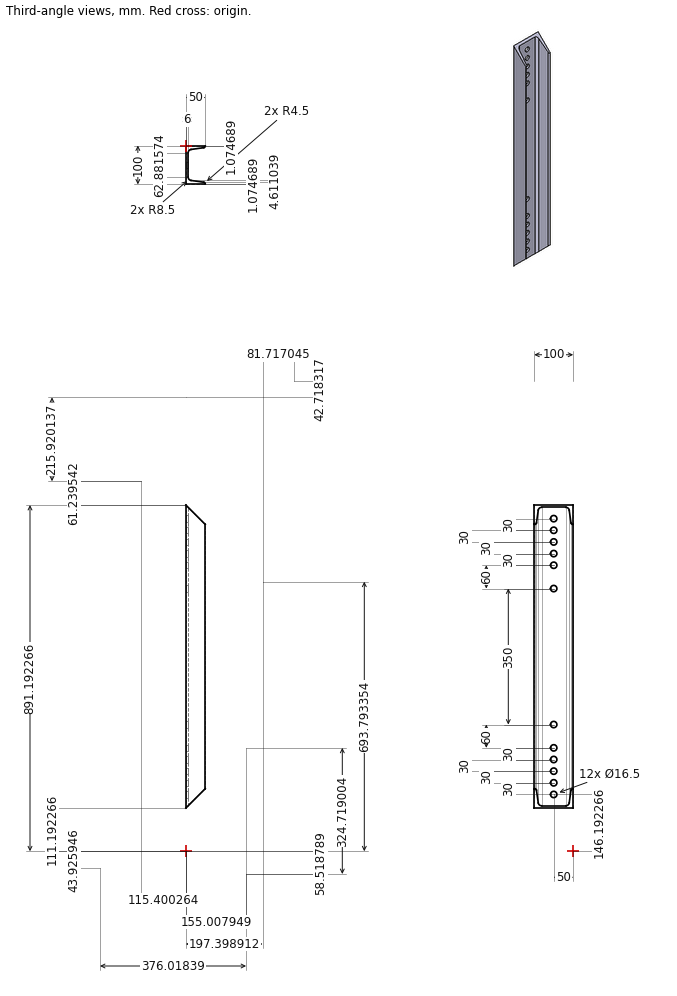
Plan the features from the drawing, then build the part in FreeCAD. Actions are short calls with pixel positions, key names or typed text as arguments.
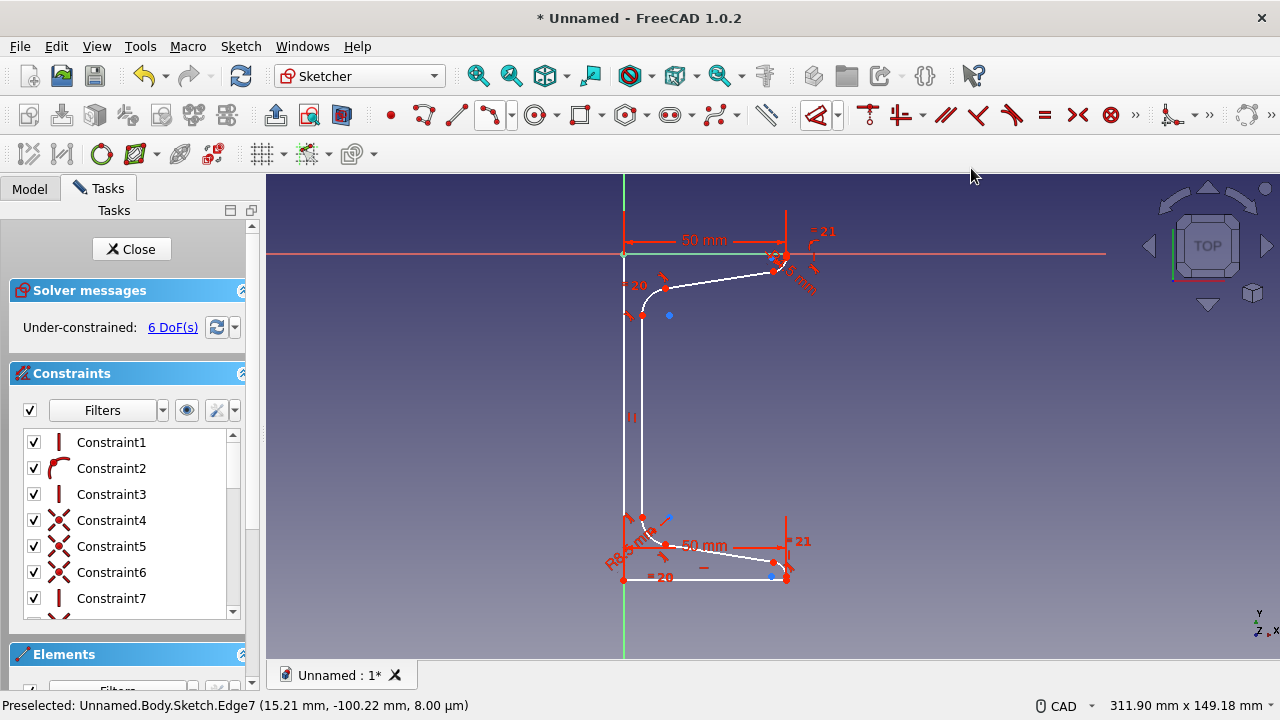
scroll(642, 518, up, 4)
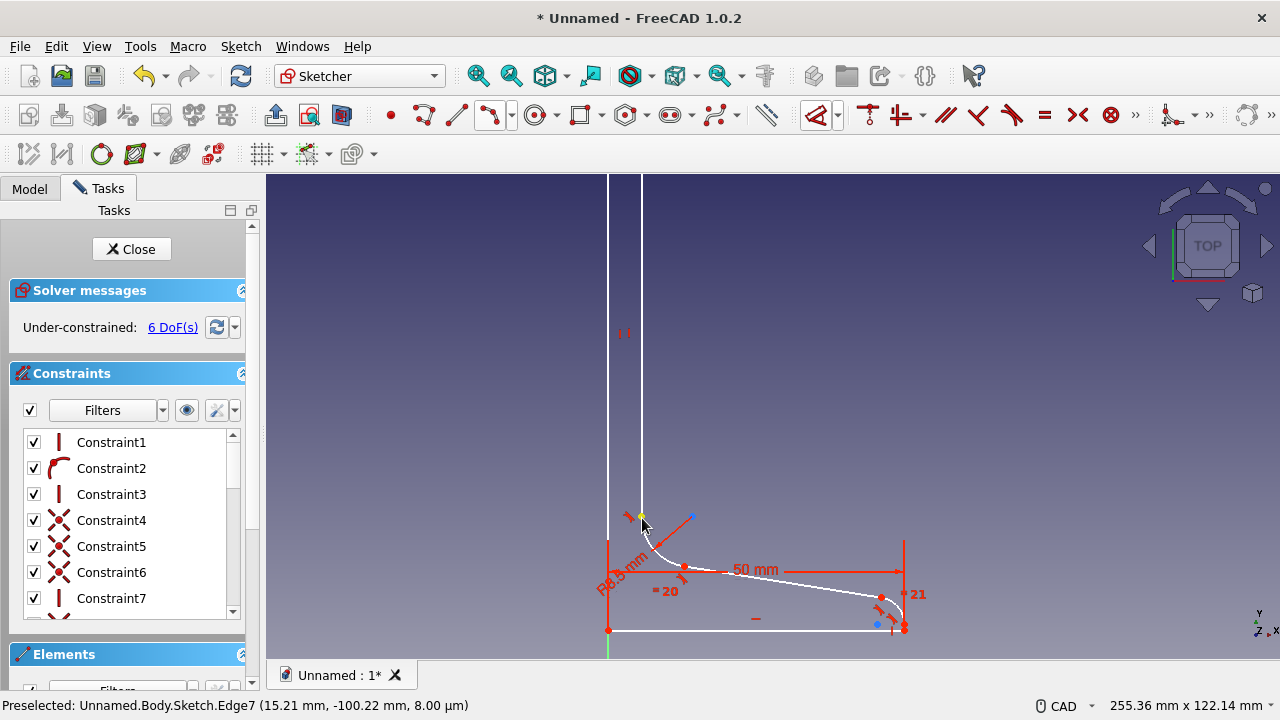
click(642, 516)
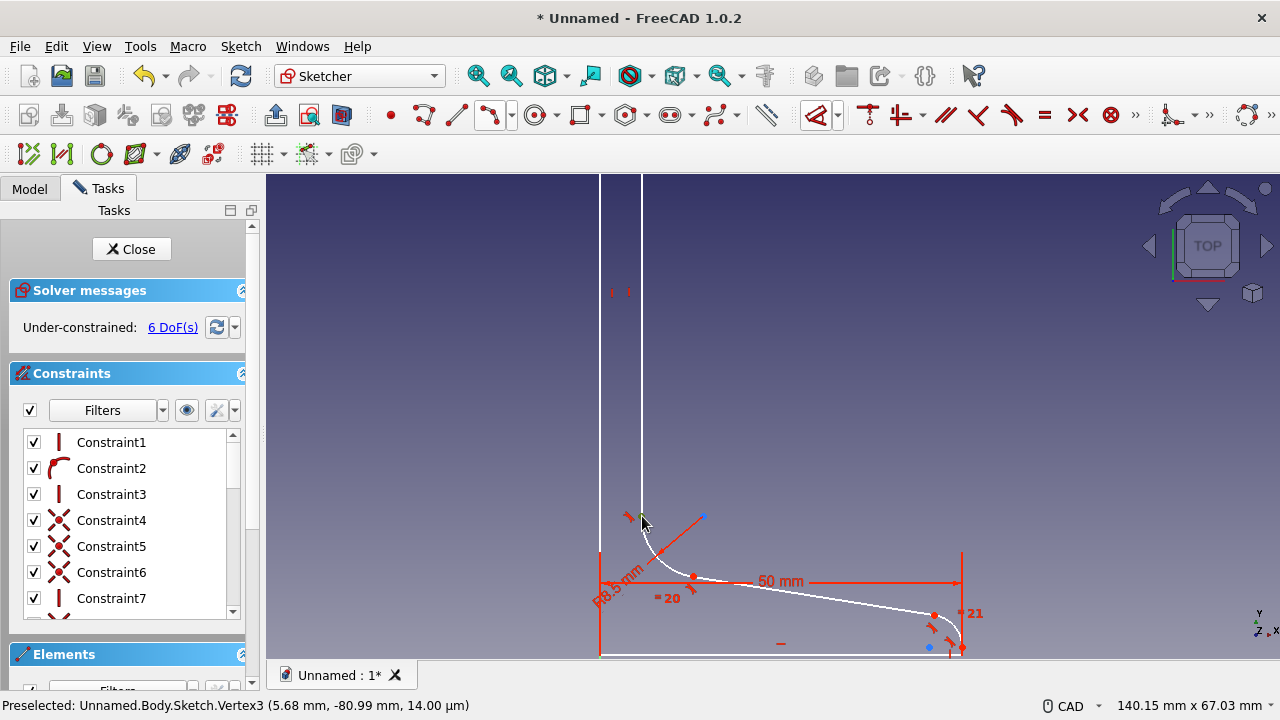
key(l)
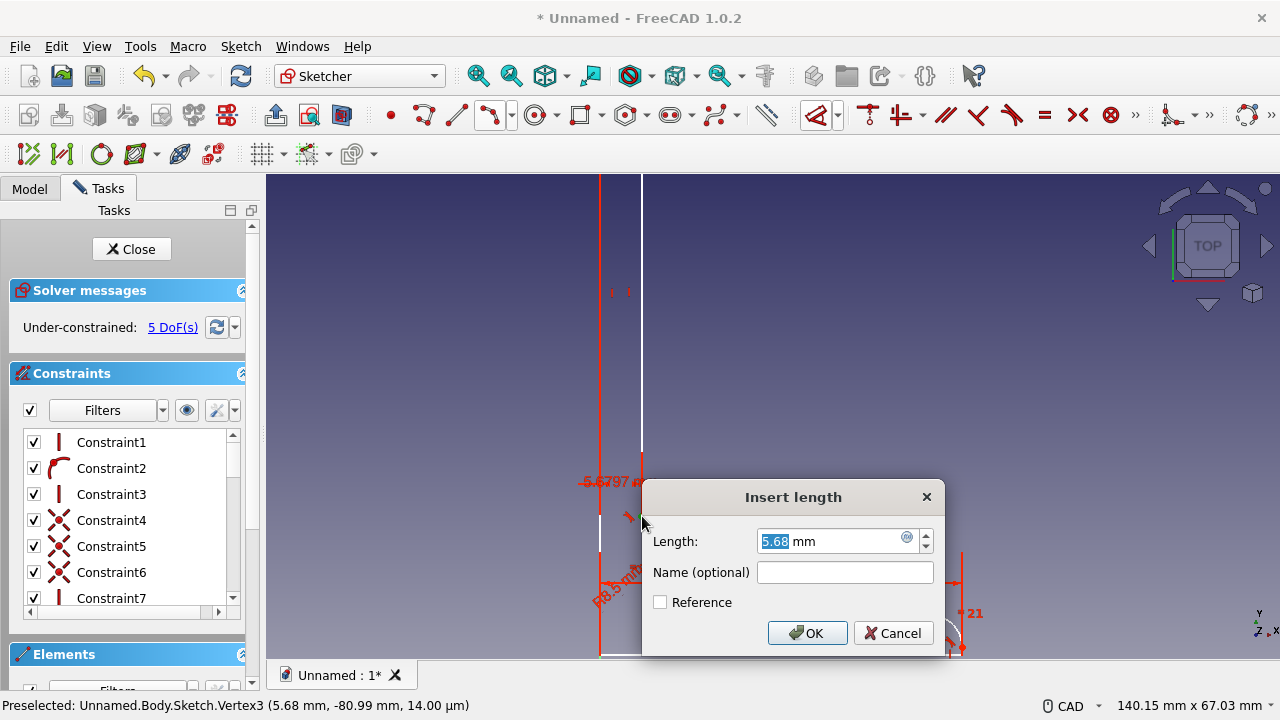
text(6)
key(Return)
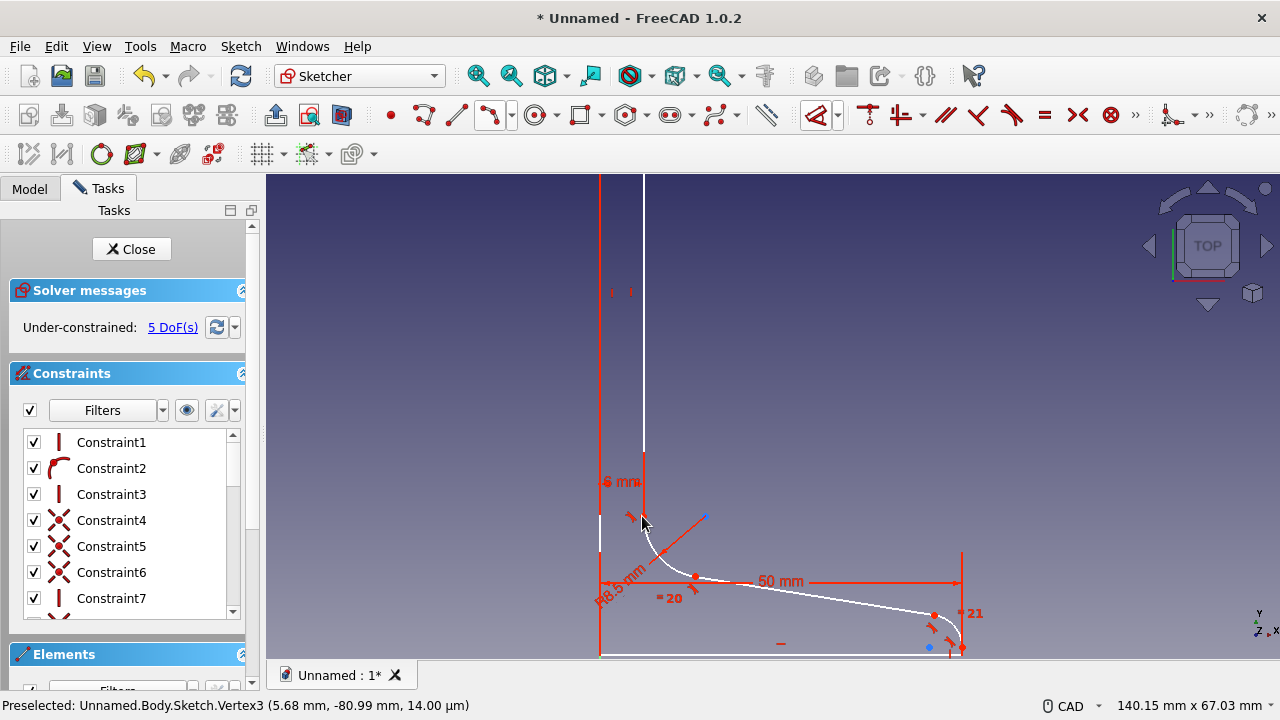
click(600, 438)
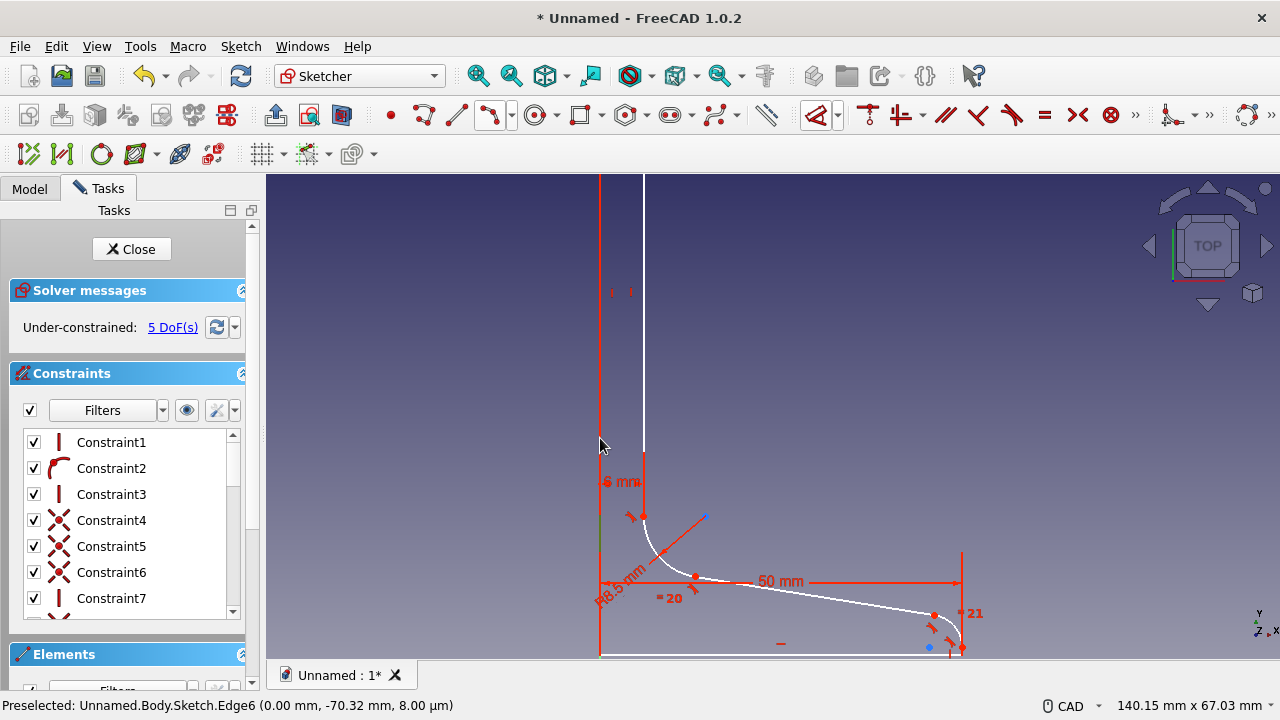
key(i)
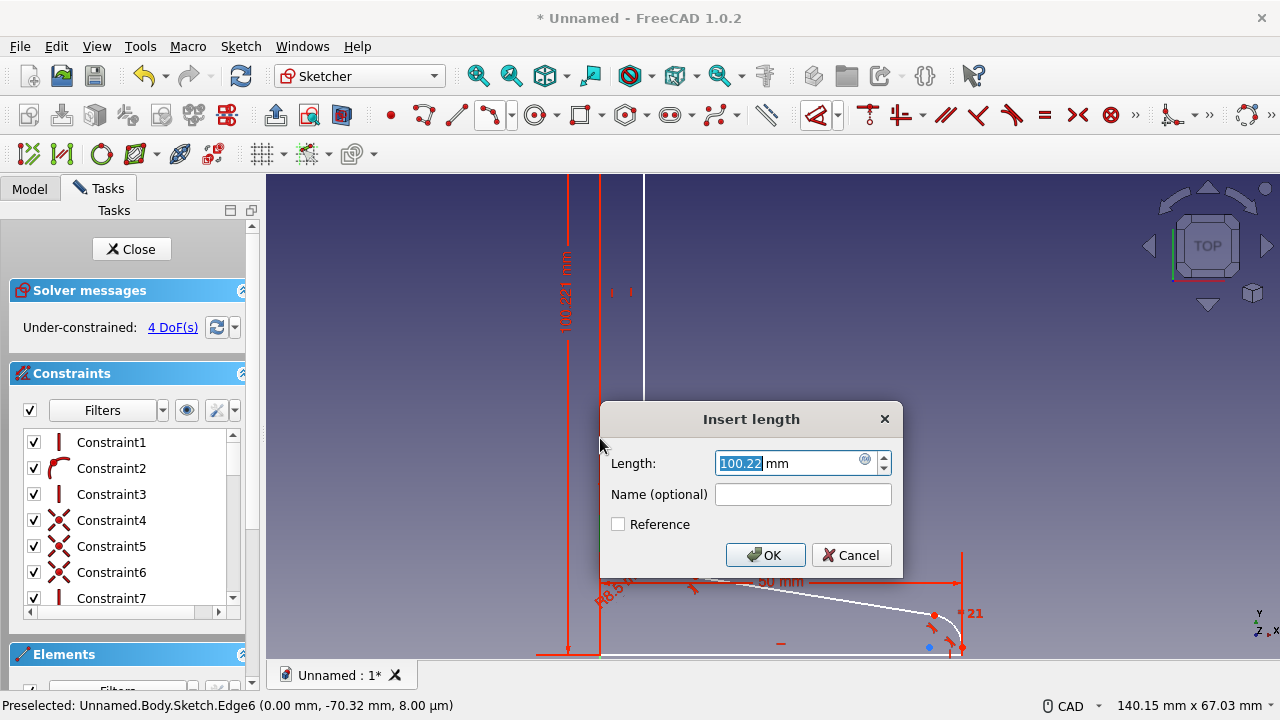
text(100)
key(Return)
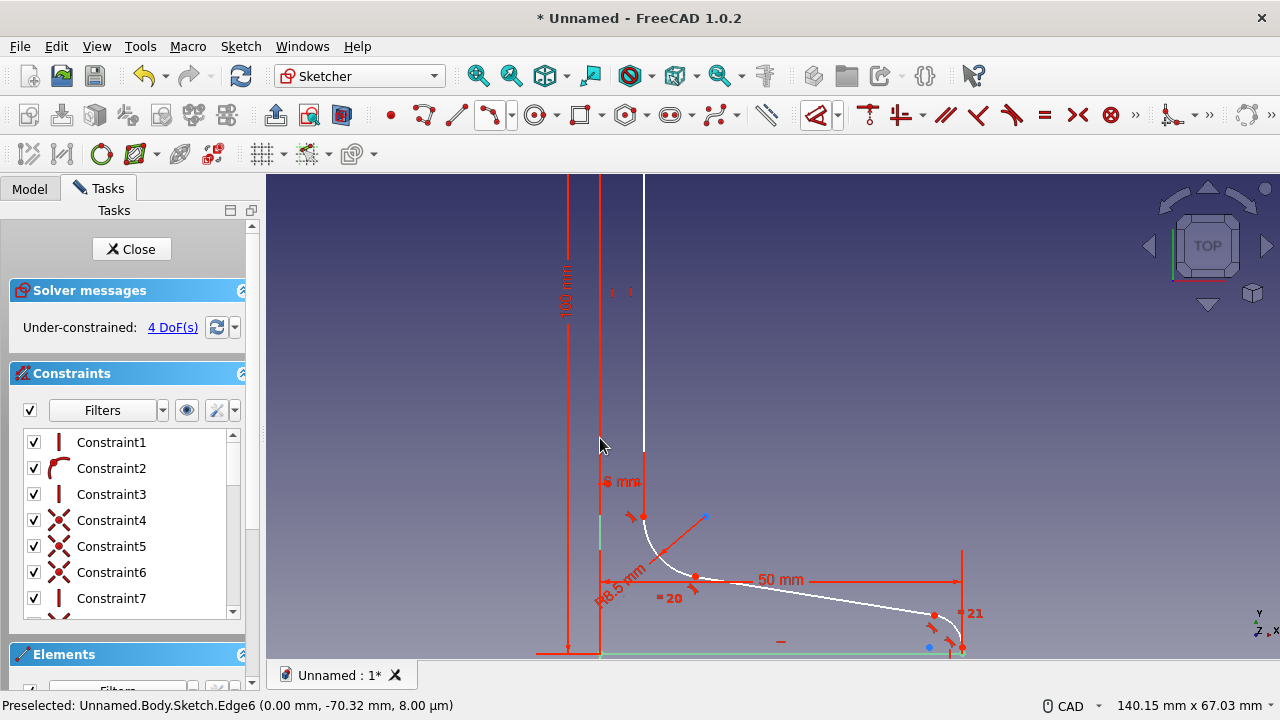
scroll(642, 518, down, 4)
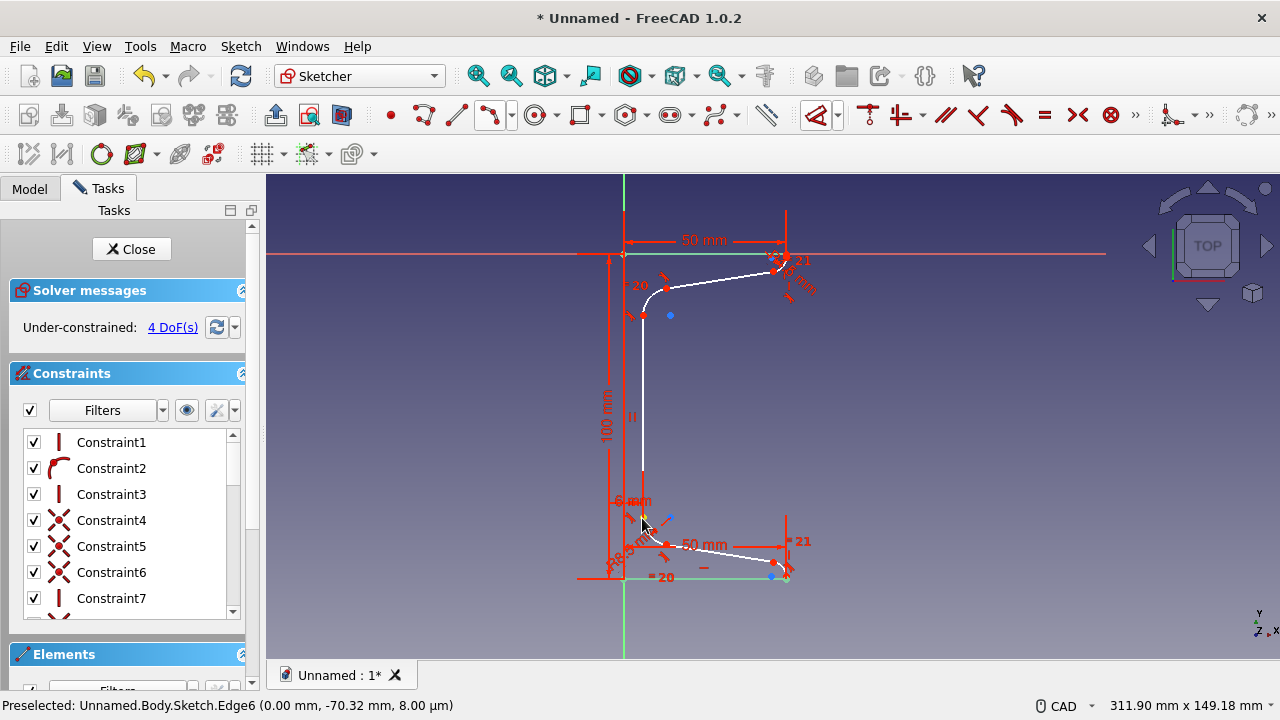
scroll(786, 256, up, 13)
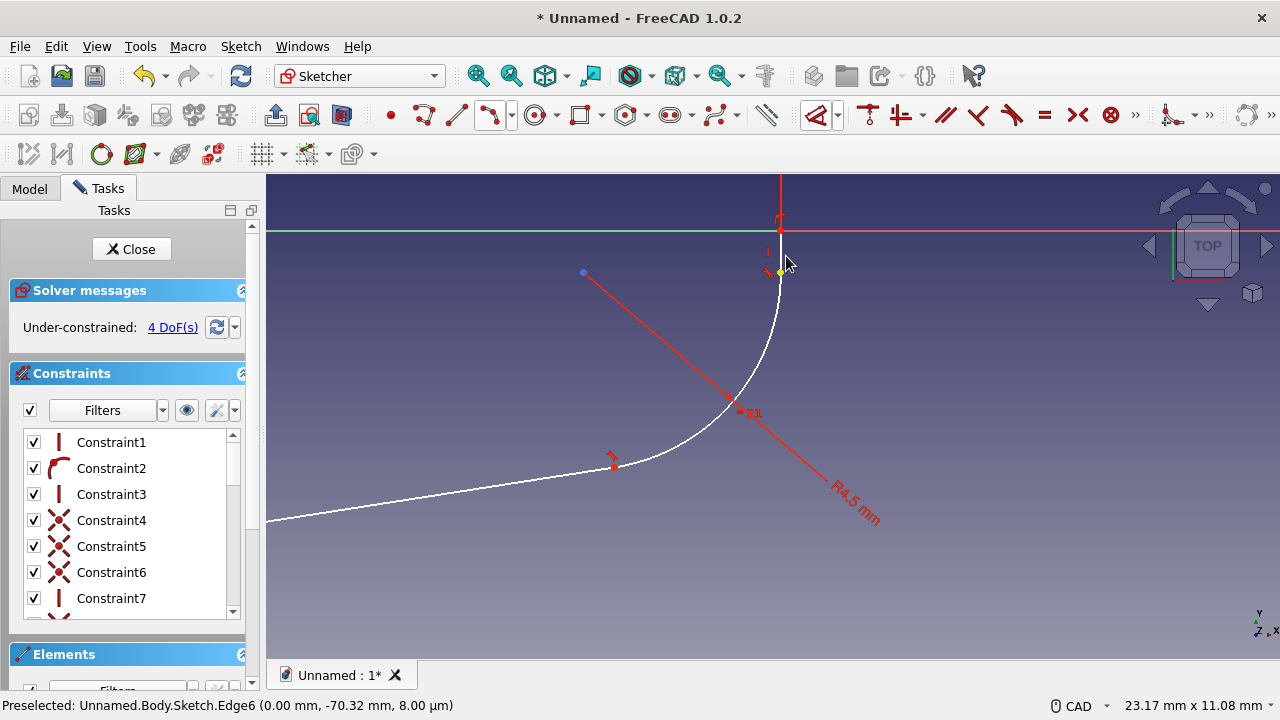
click(781, 252)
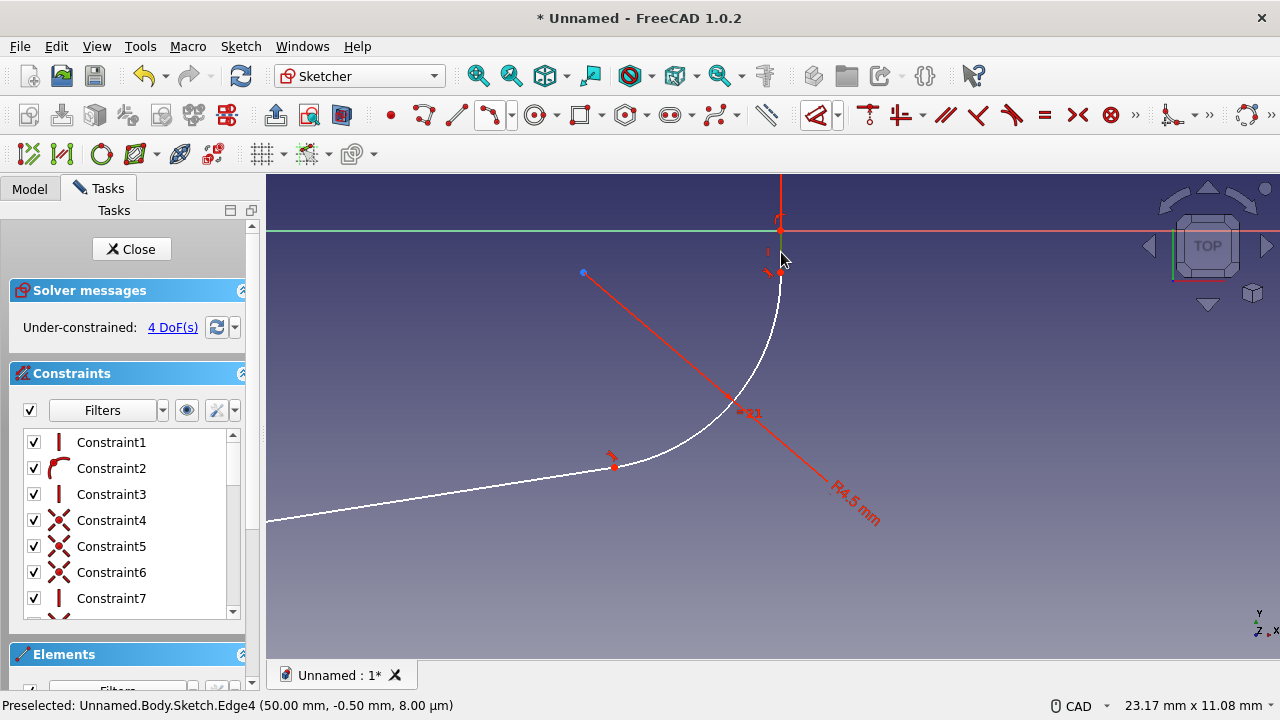
click(838, 116)